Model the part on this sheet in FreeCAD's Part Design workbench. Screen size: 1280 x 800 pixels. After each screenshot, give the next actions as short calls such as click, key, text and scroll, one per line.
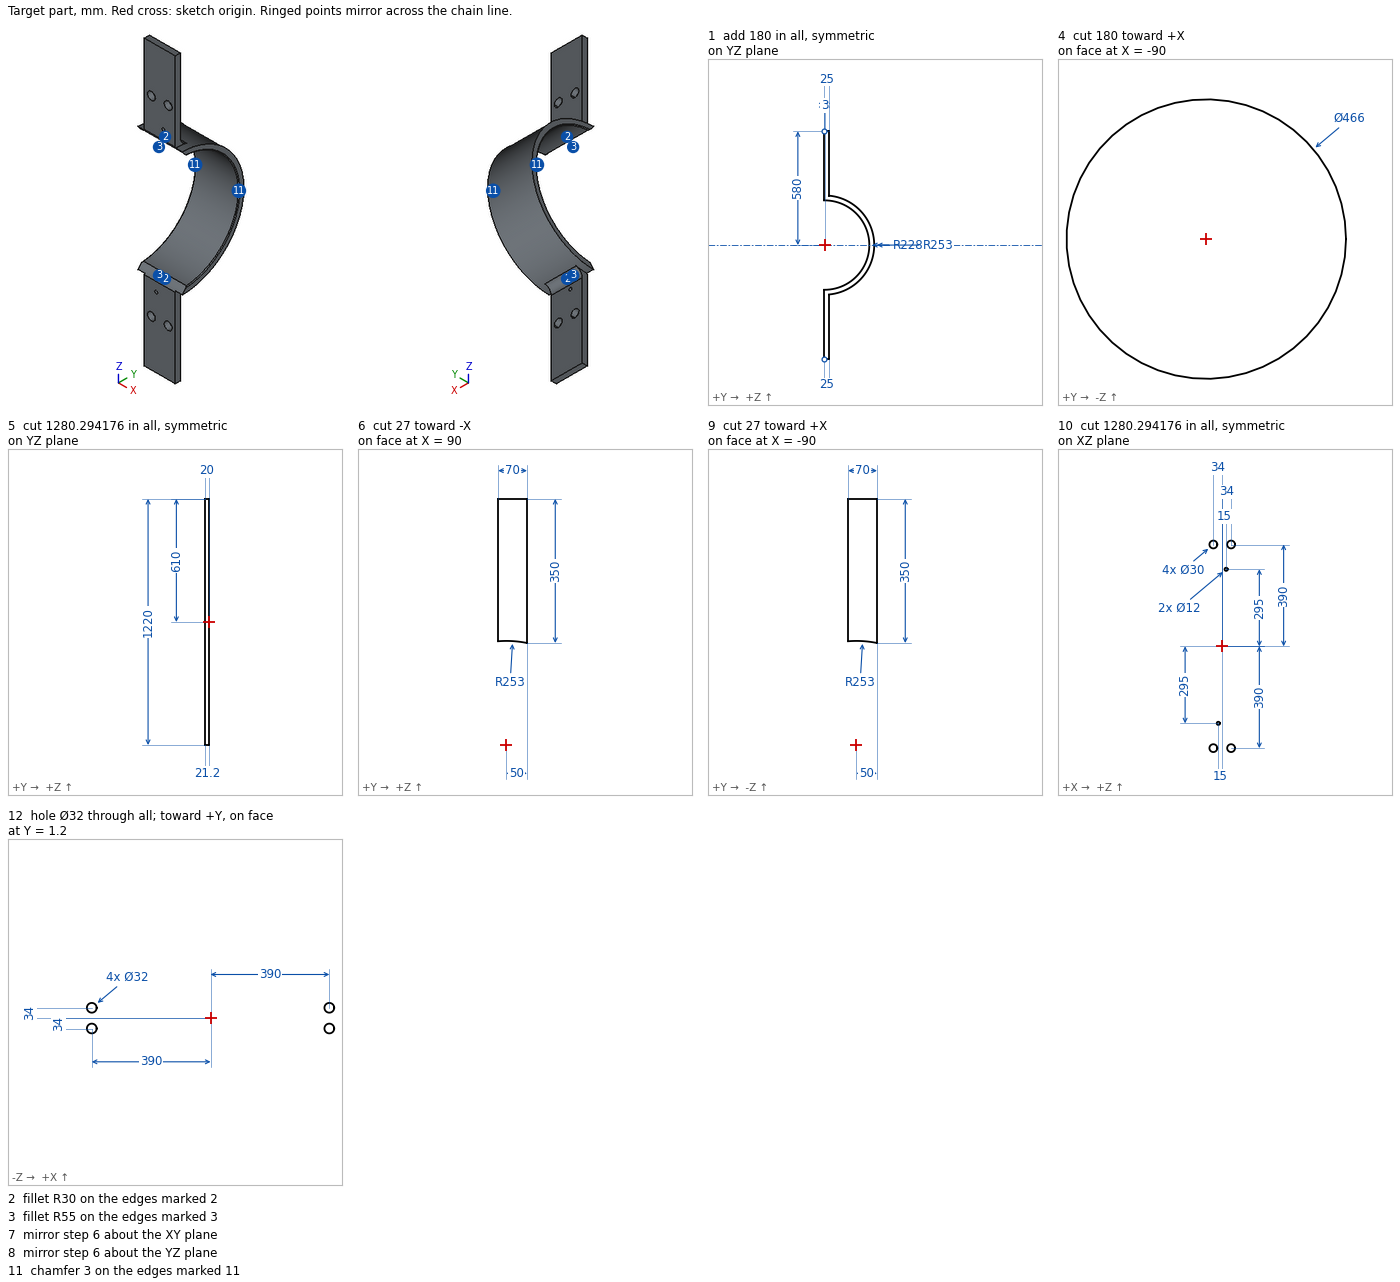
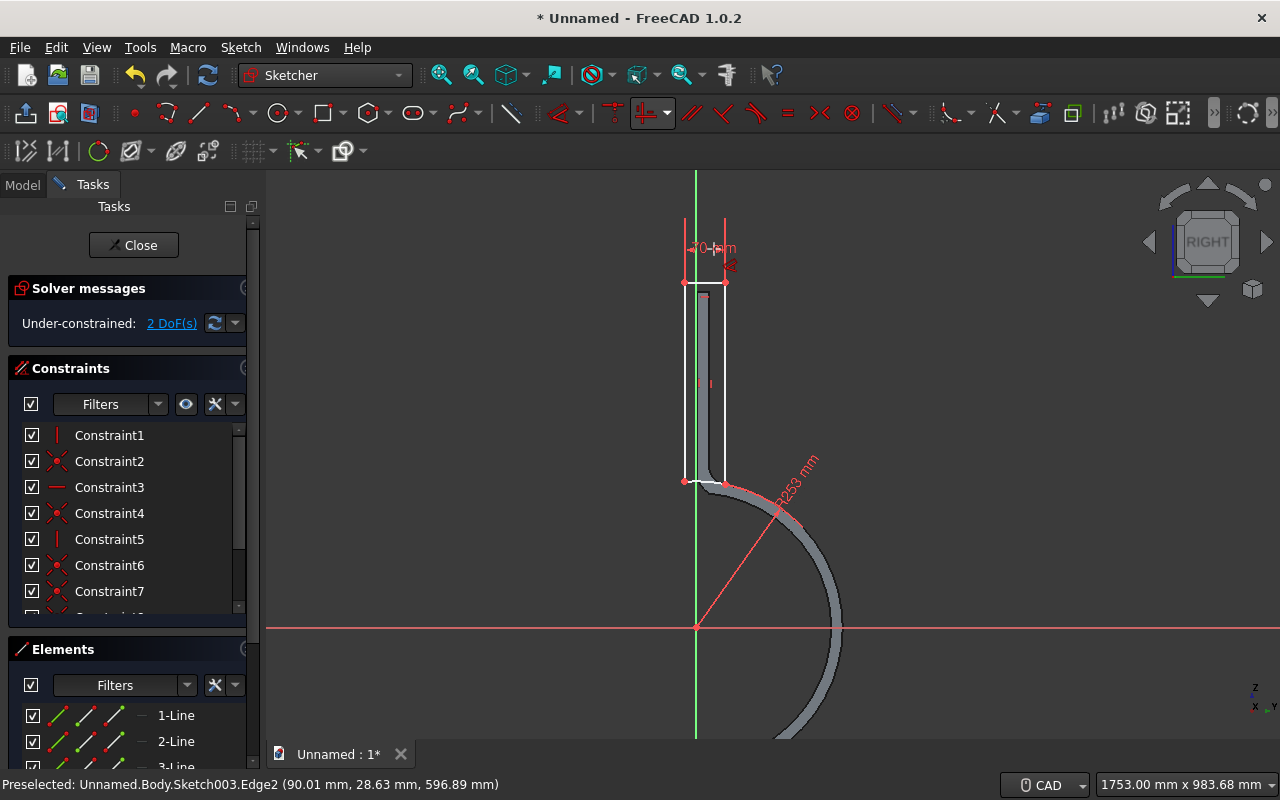
click(725, 424)
click(759, 383)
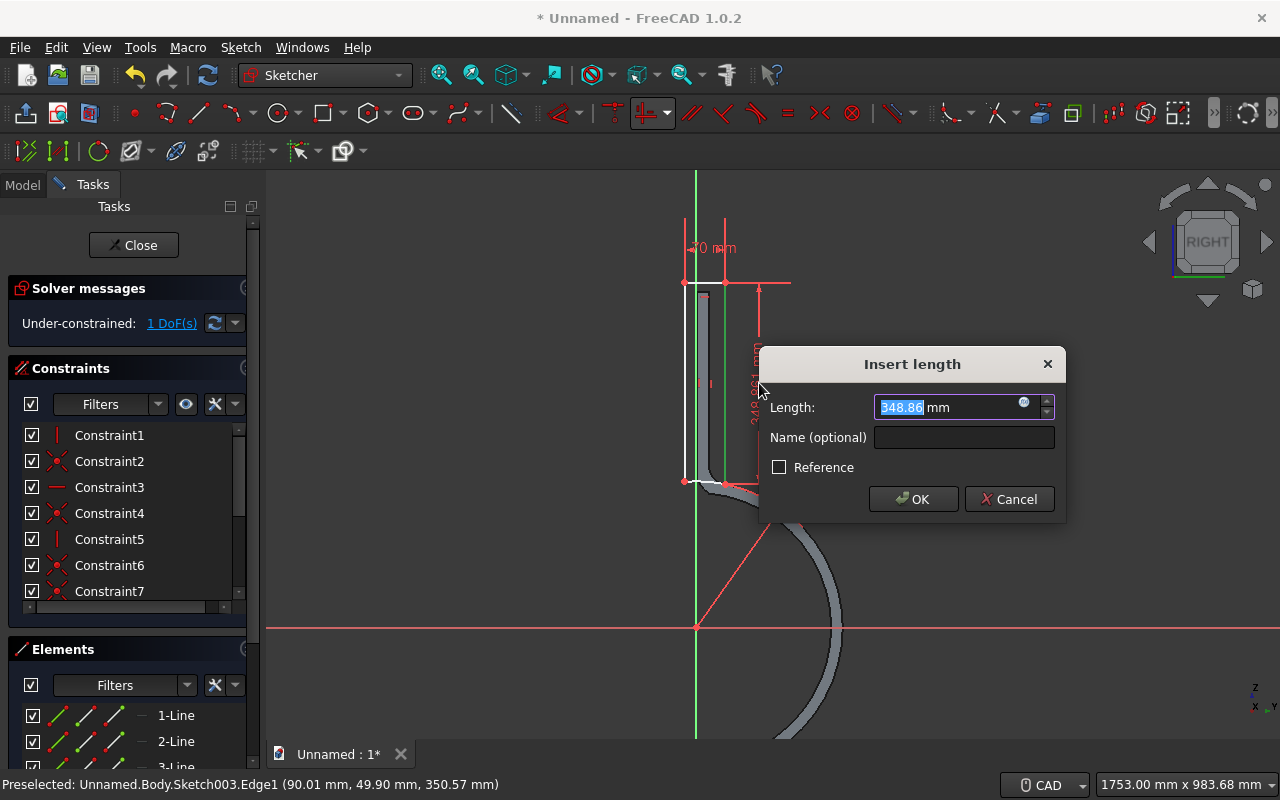
text(350)
key(Return)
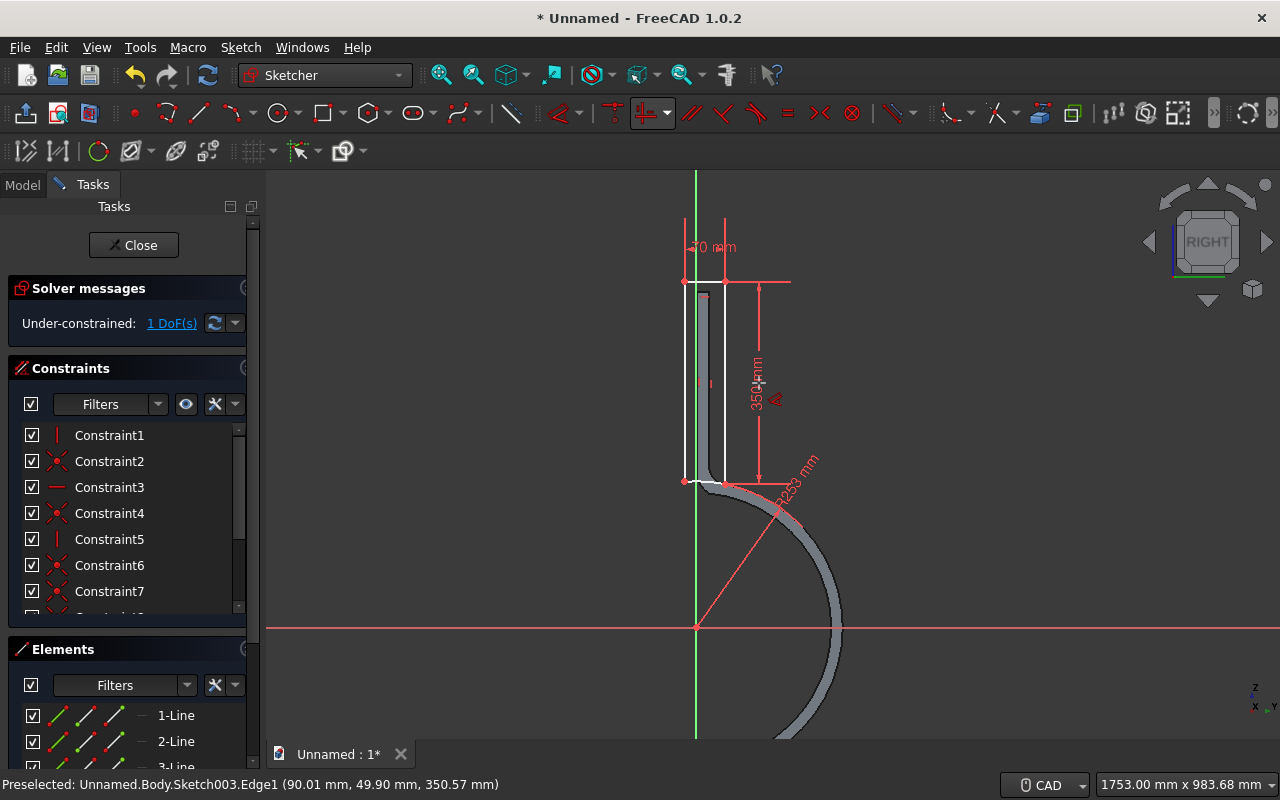
scroll(725, 484, up, 2)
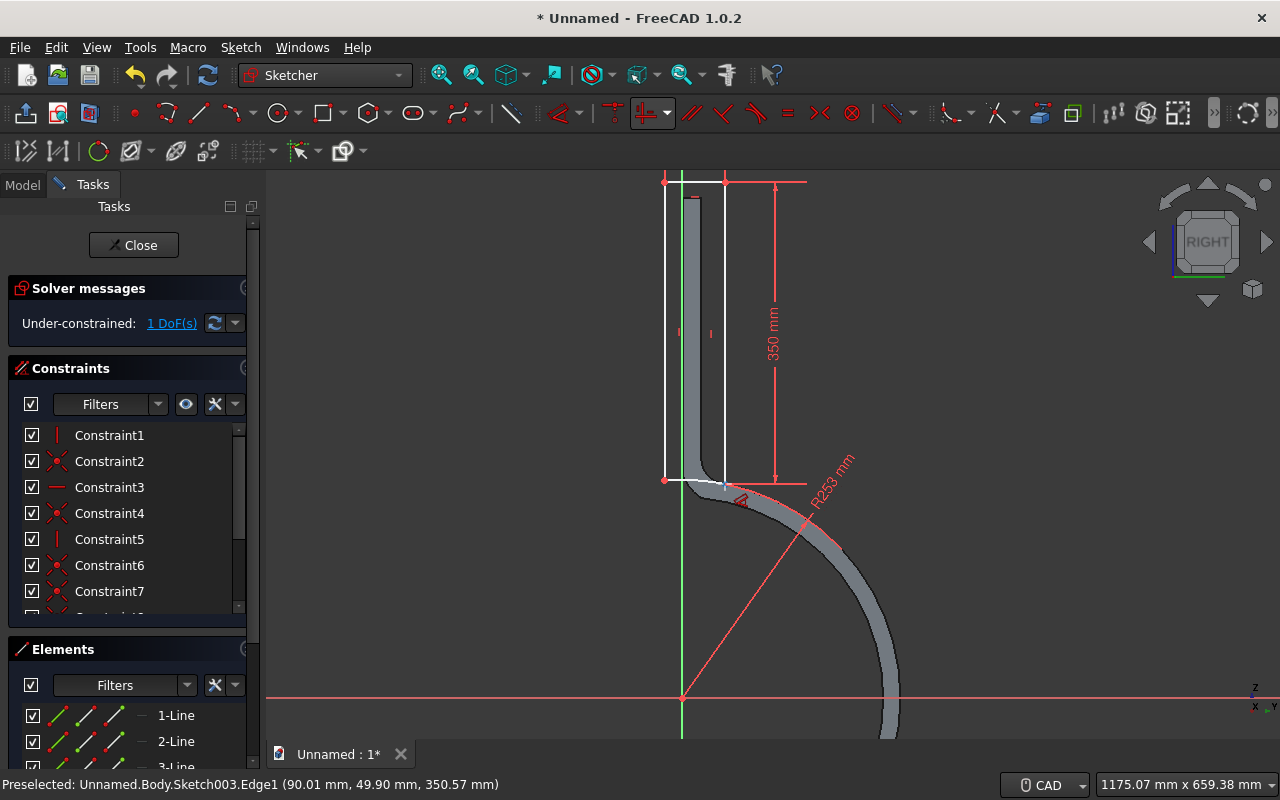
click(725, 484)
click(704, 450)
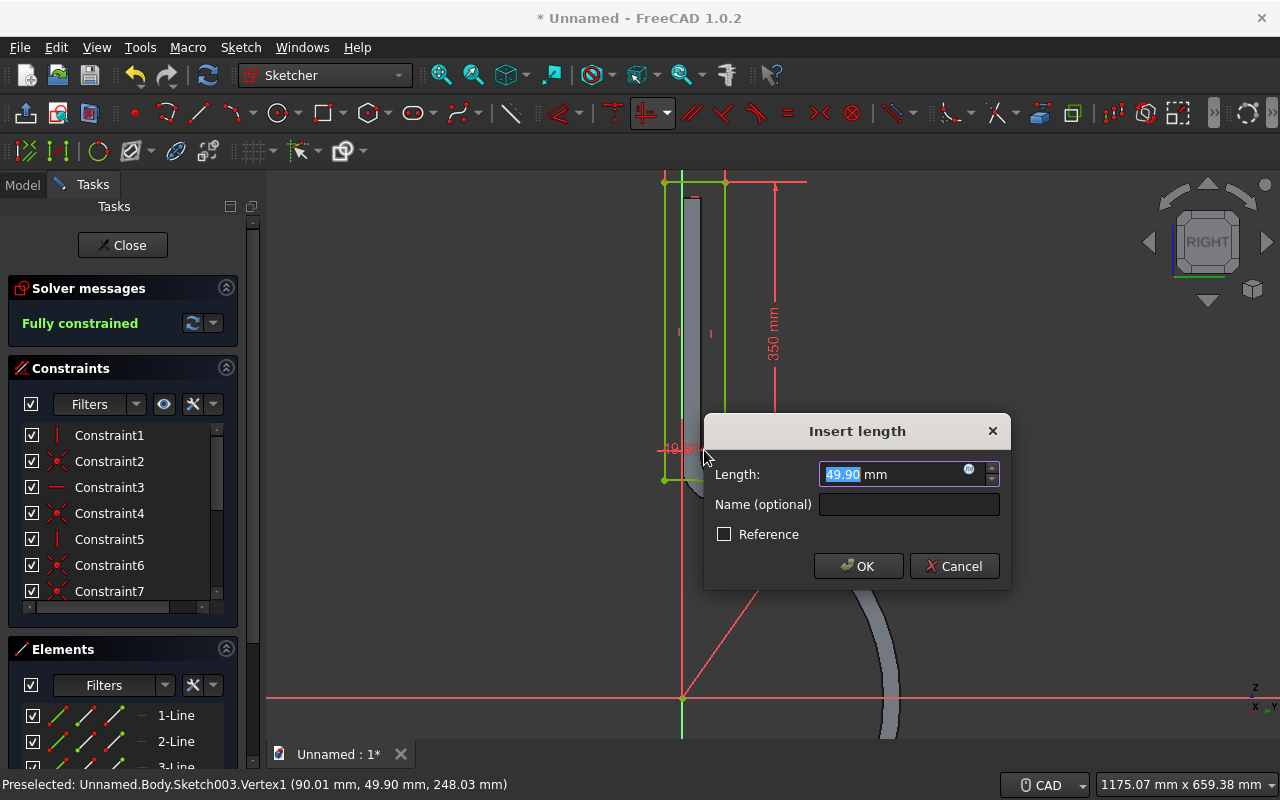
text(50)
key(Return)
key(Escape)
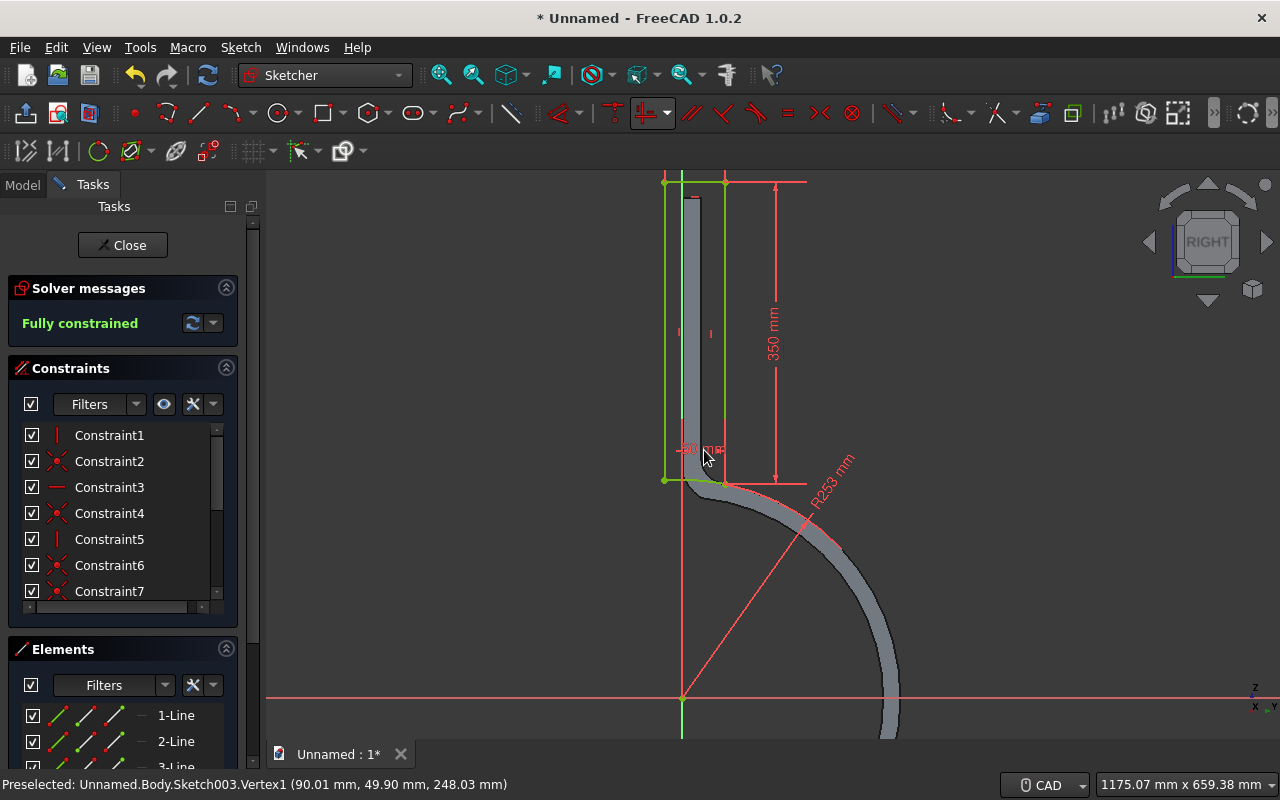
click(123, 245)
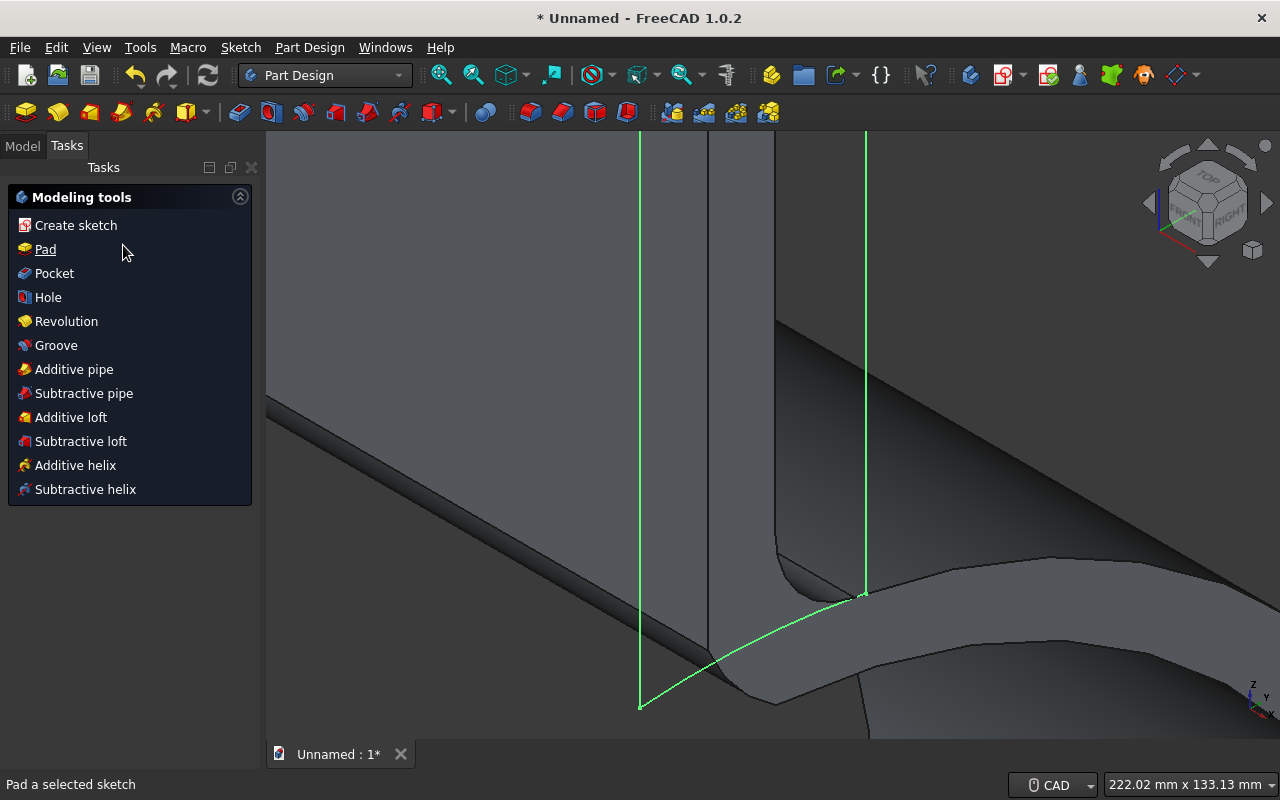
click(240, 112)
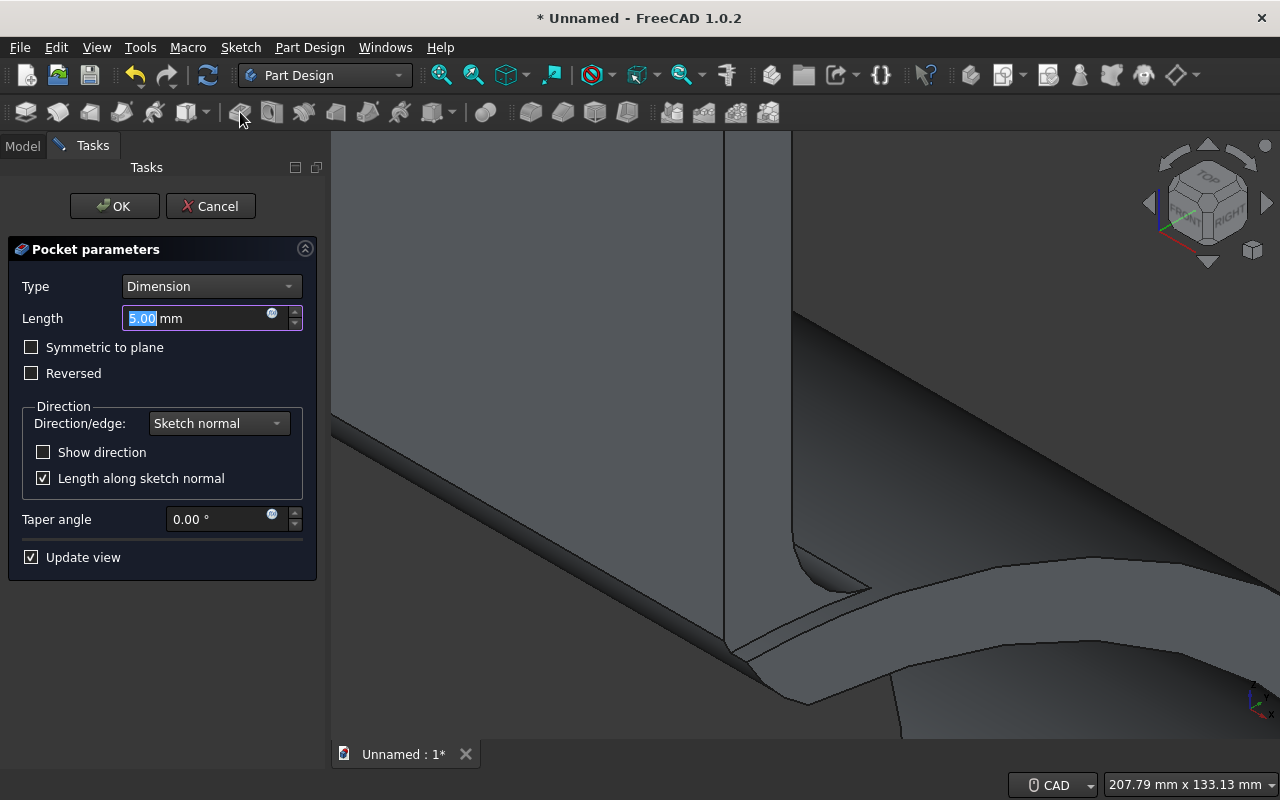
text(27)
key(Tab)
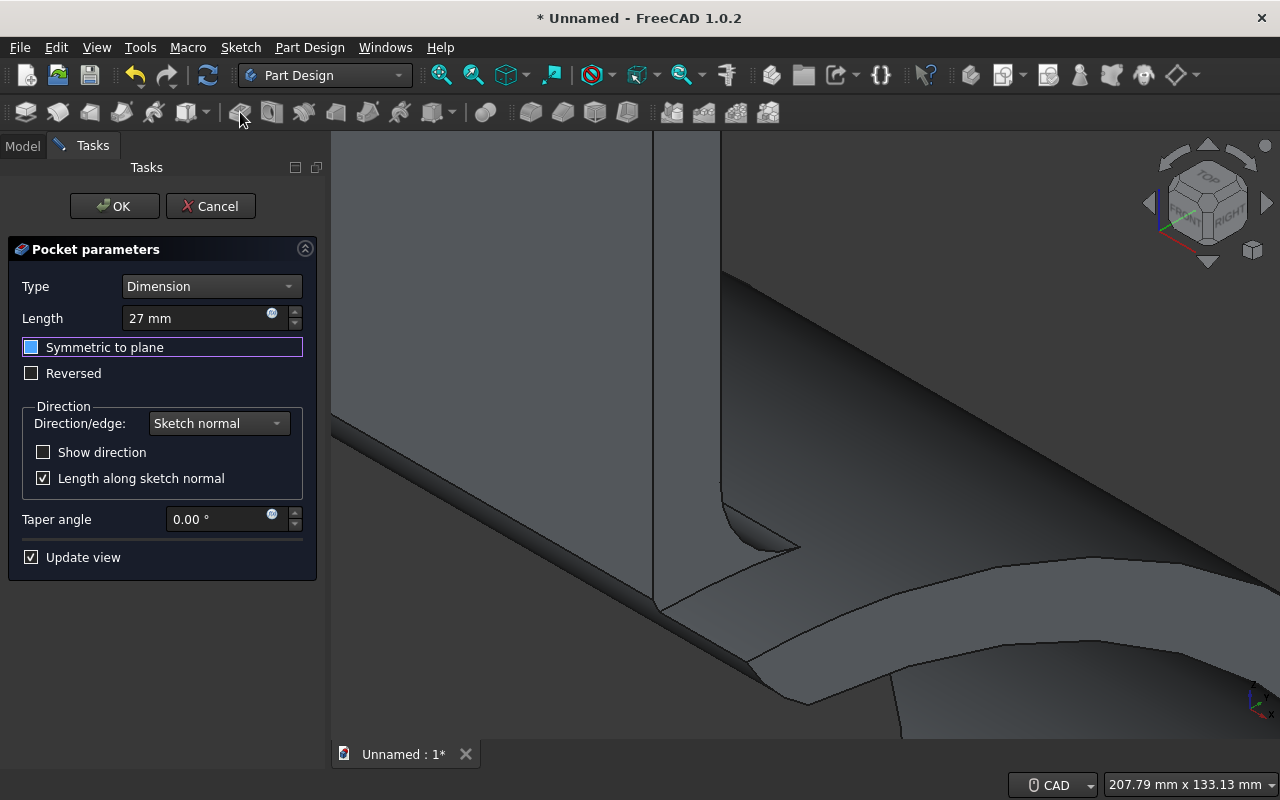
click(115, 206)